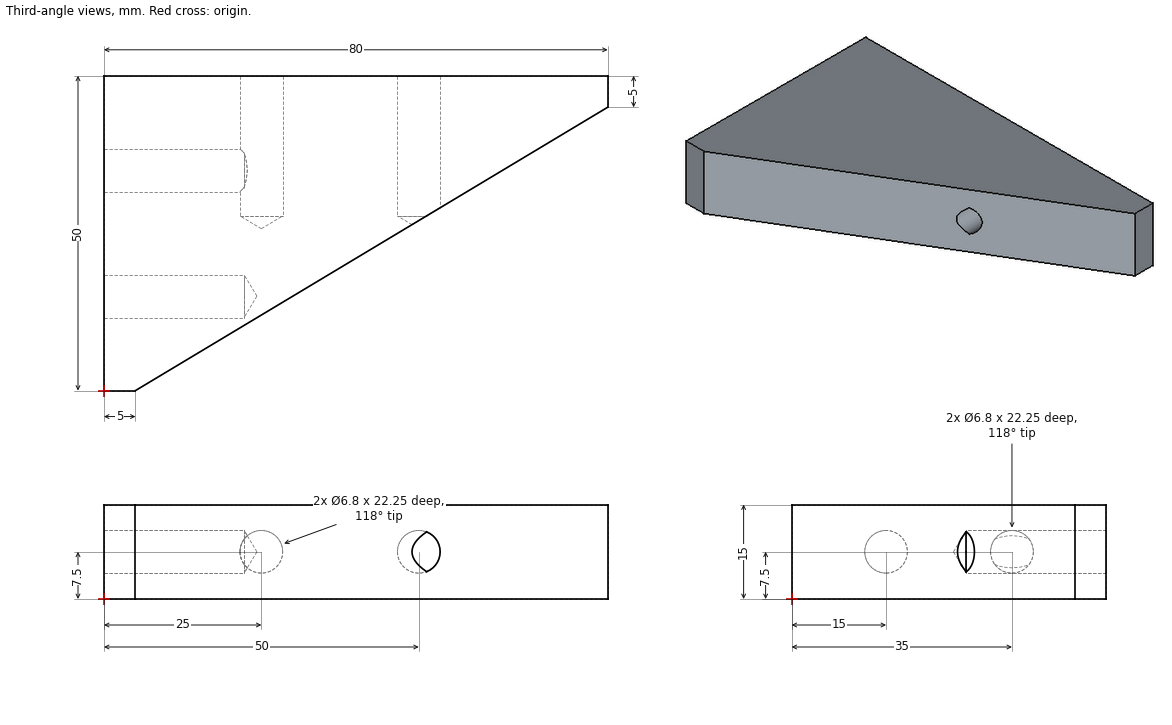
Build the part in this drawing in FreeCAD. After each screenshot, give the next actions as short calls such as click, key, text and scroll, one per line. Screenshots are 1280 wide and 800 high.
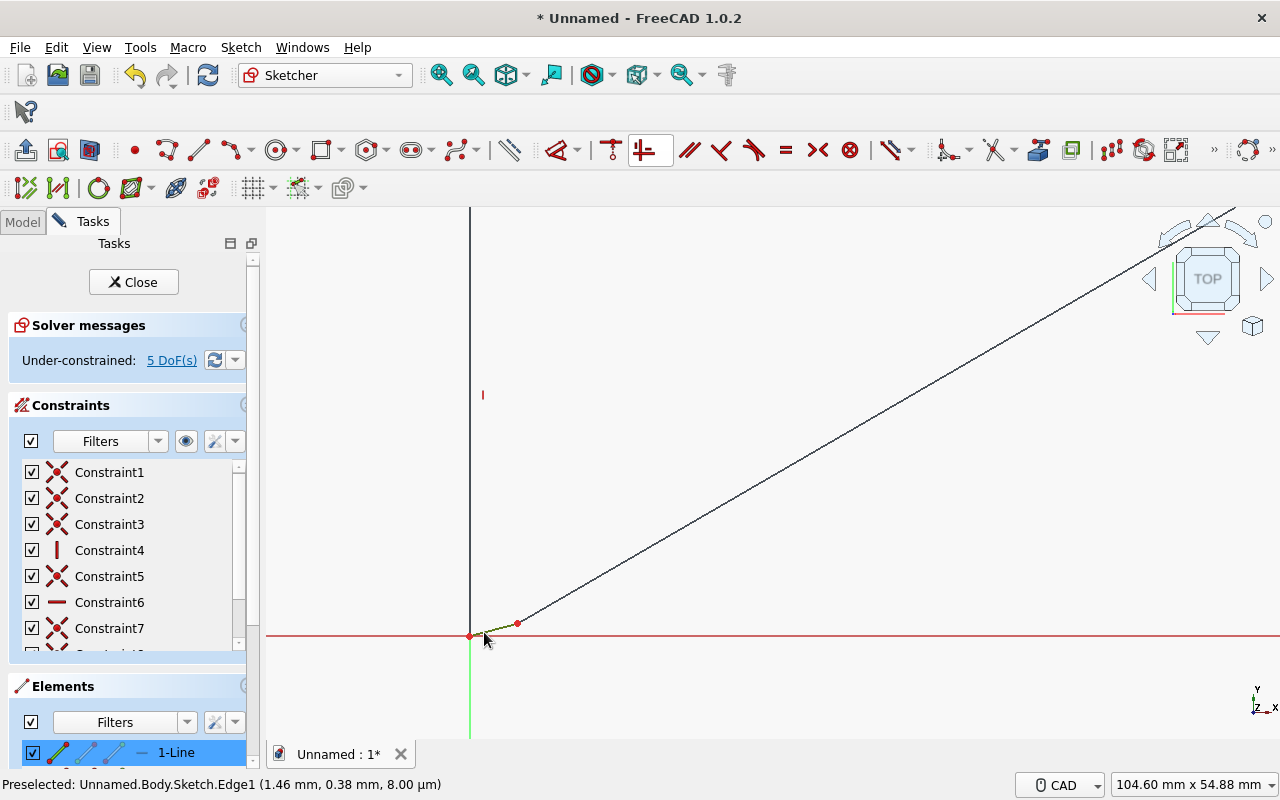
key(h)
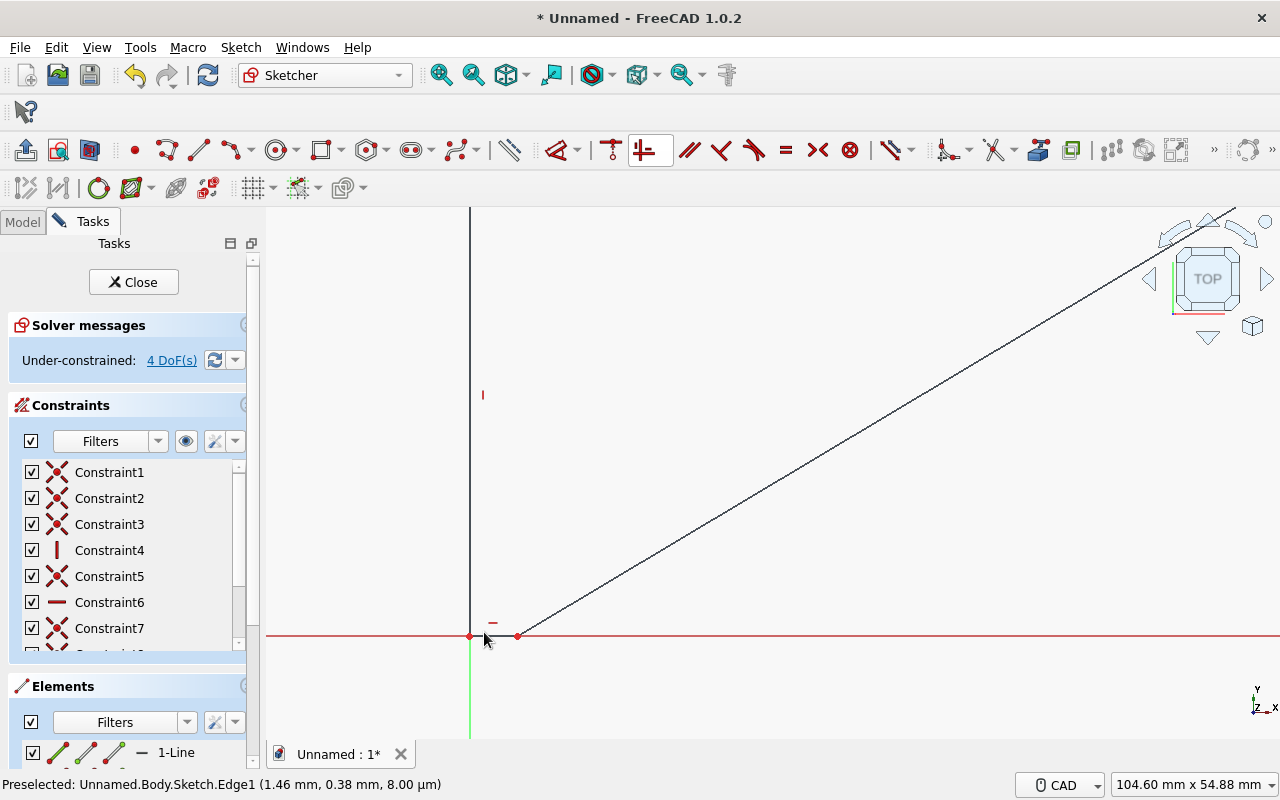
click(556, 150)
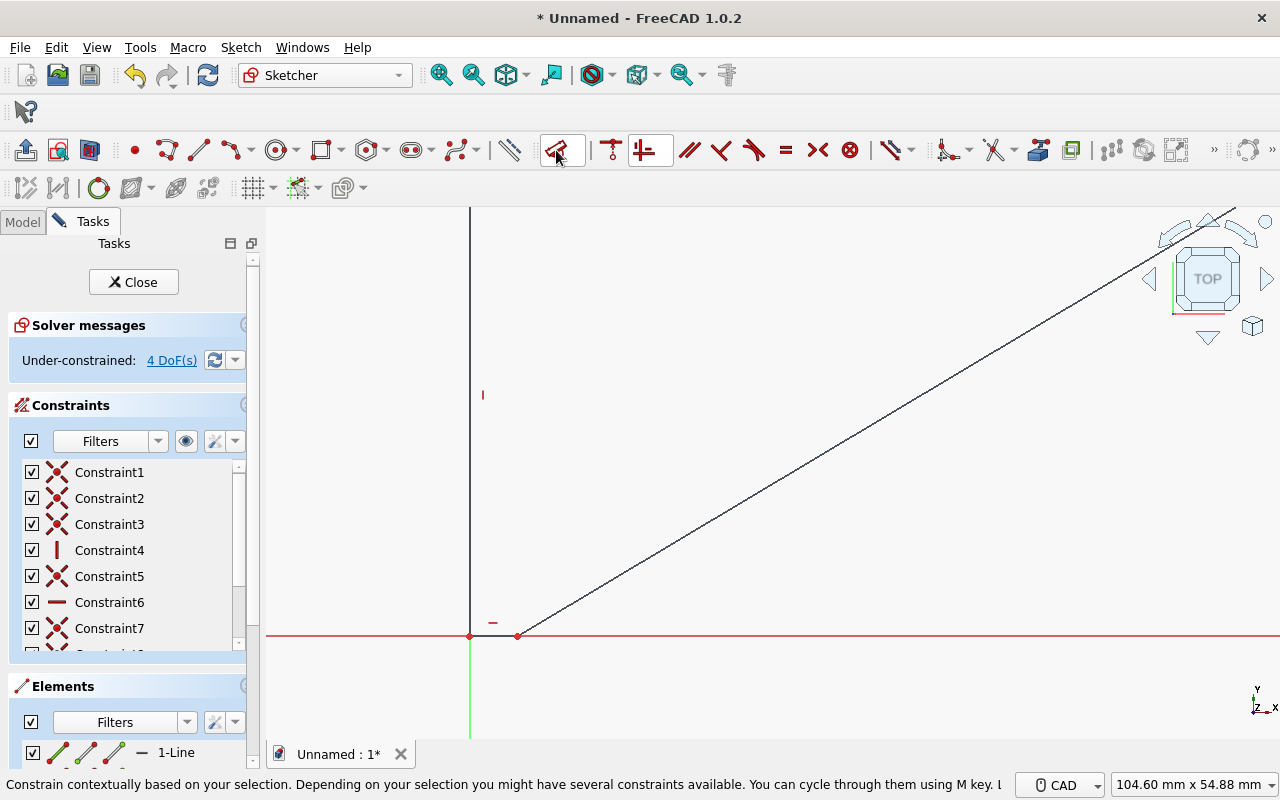
click(484, 636)
click(494, 670)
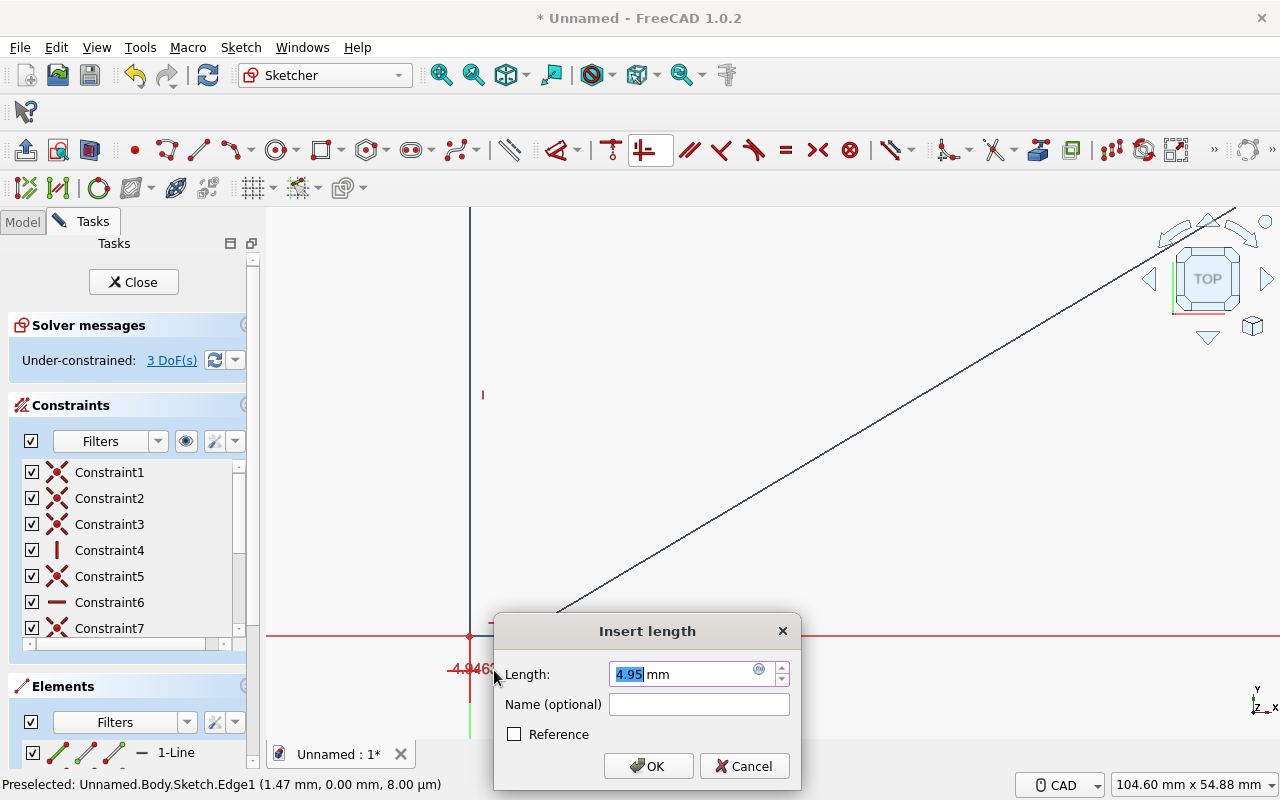
text(5)
key(Return)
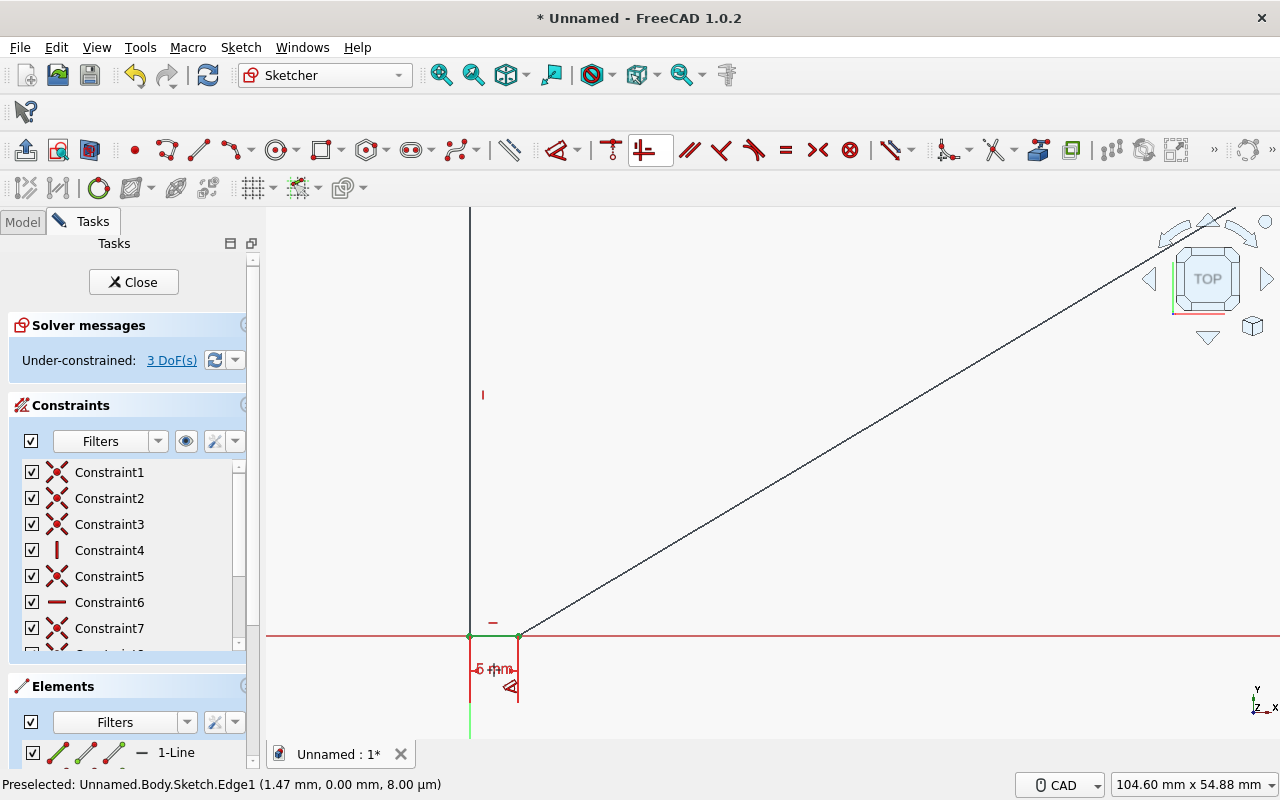
scroll(393, 634, down, 2)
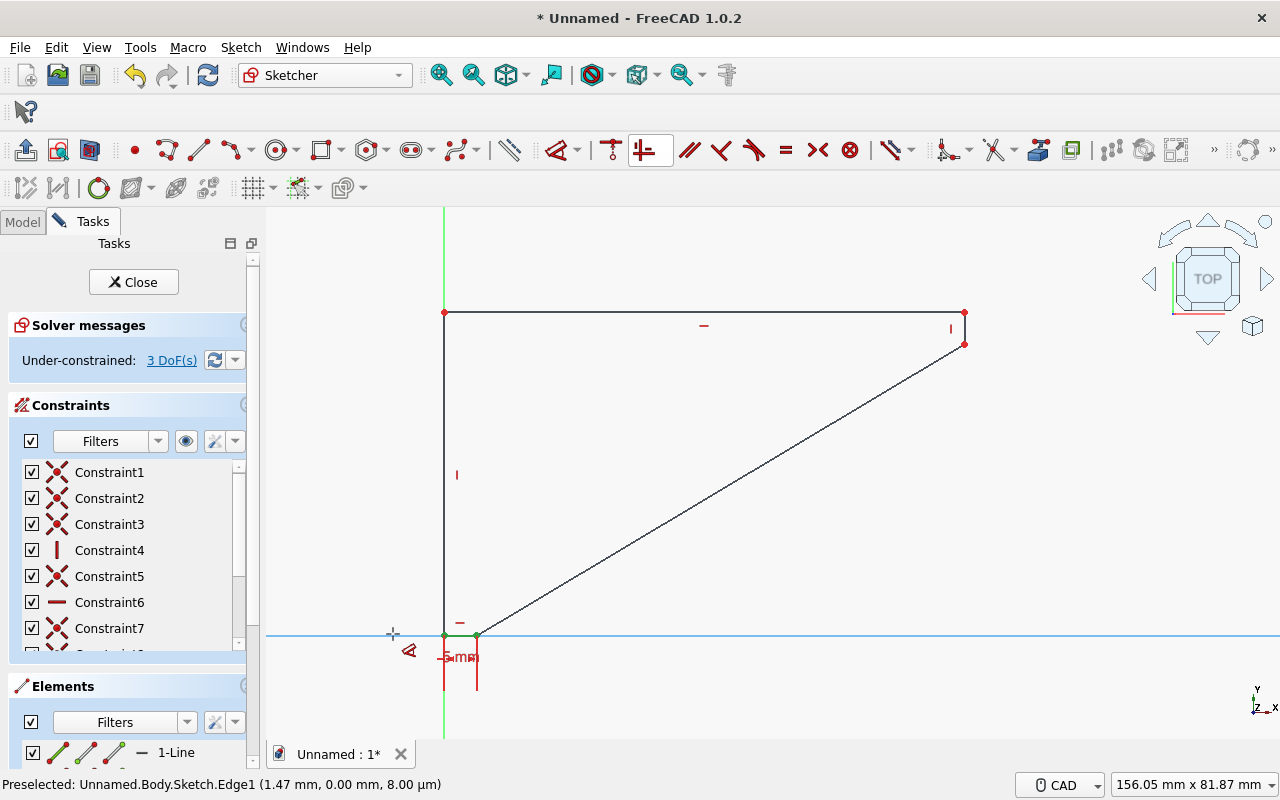
scroll(965, 335, up, 2)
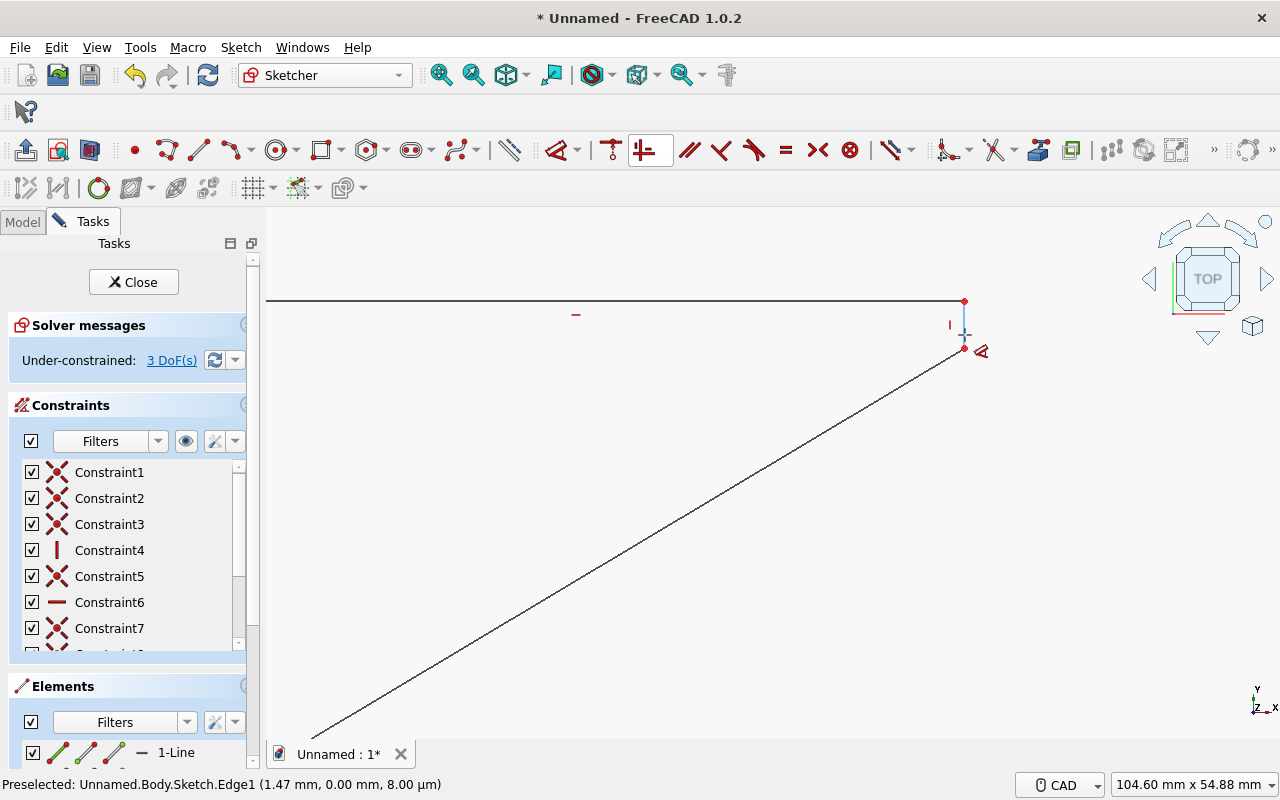
click(964, 334)
click(998, 325)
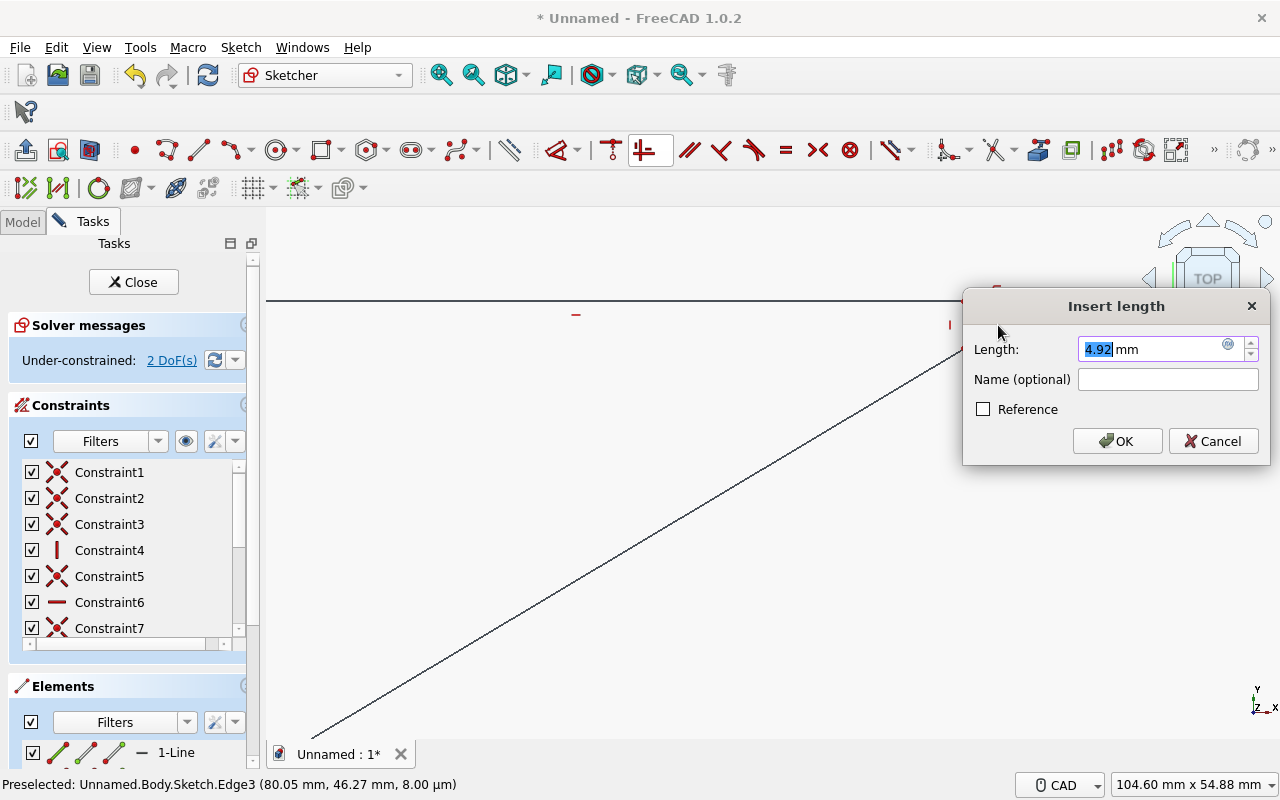
text(5)
key(Return)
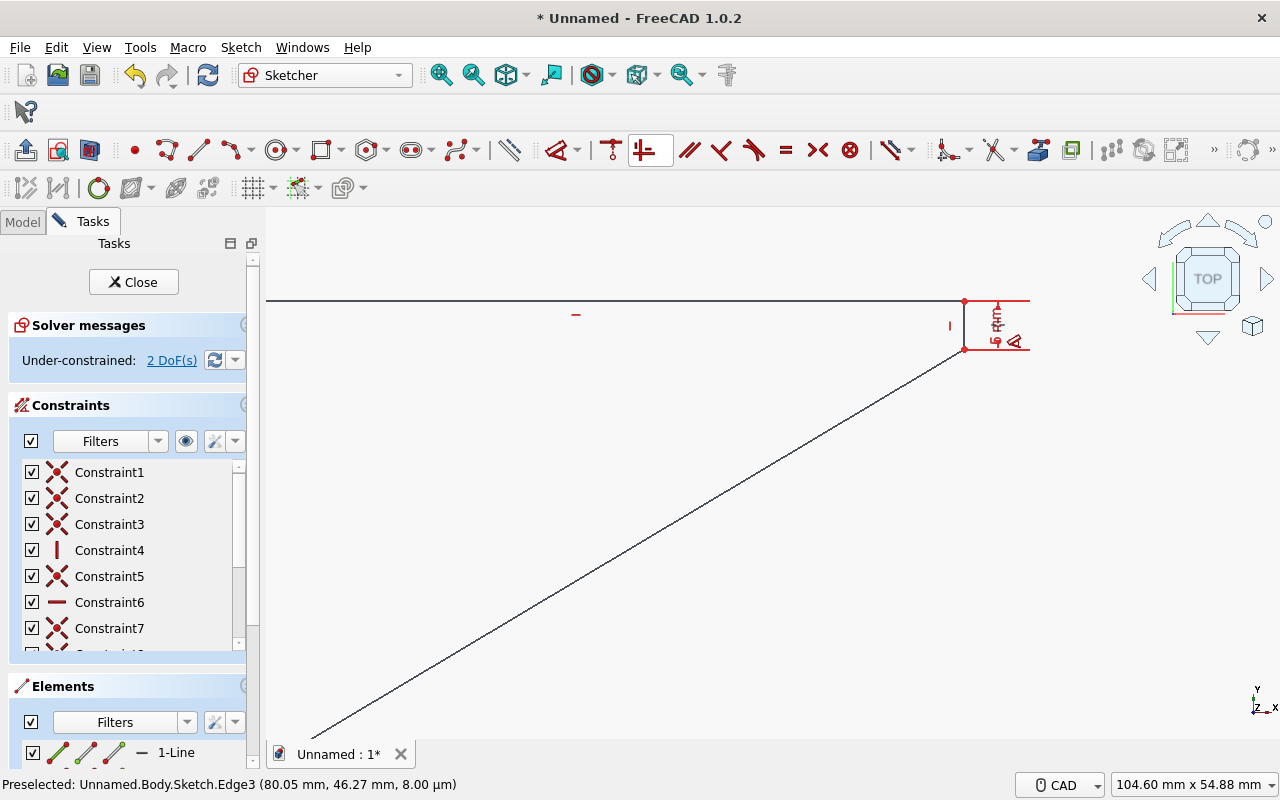
click(731, 301)
click(629, 267)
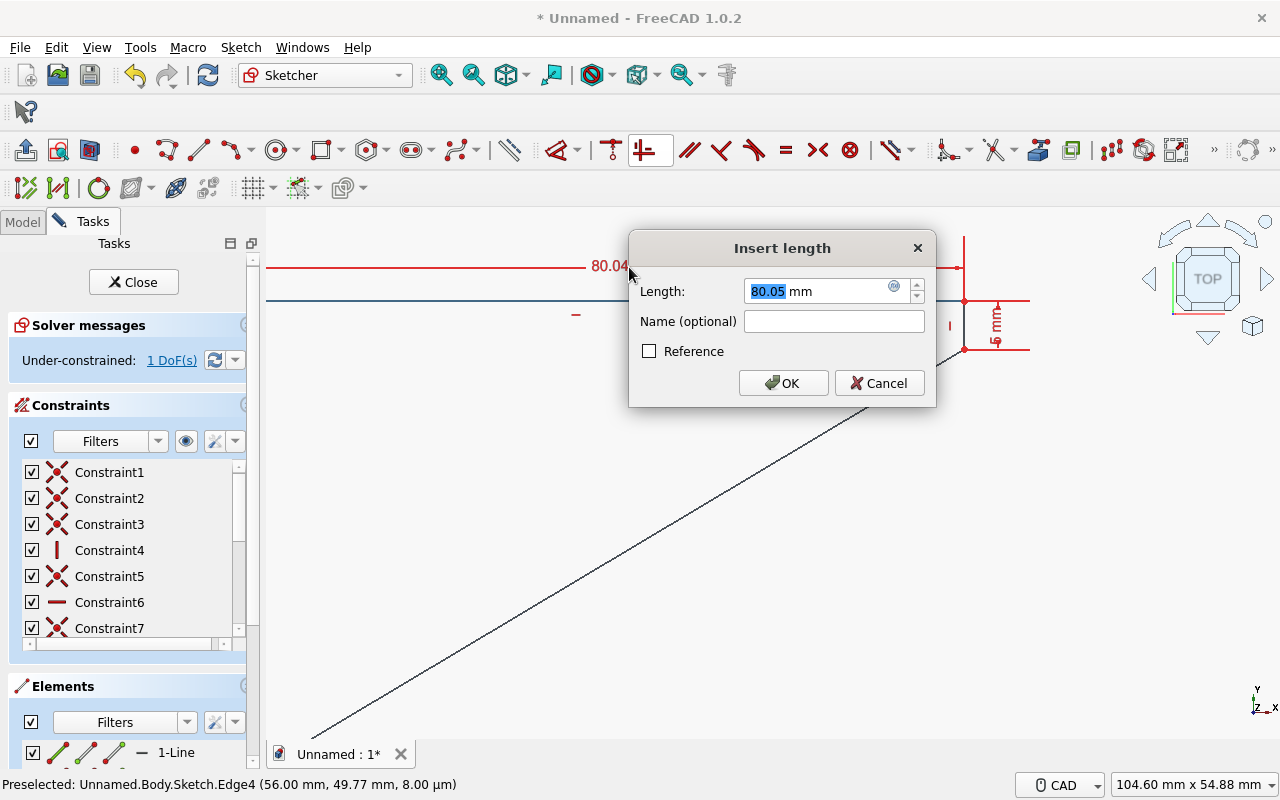
text(80)
key(Return)